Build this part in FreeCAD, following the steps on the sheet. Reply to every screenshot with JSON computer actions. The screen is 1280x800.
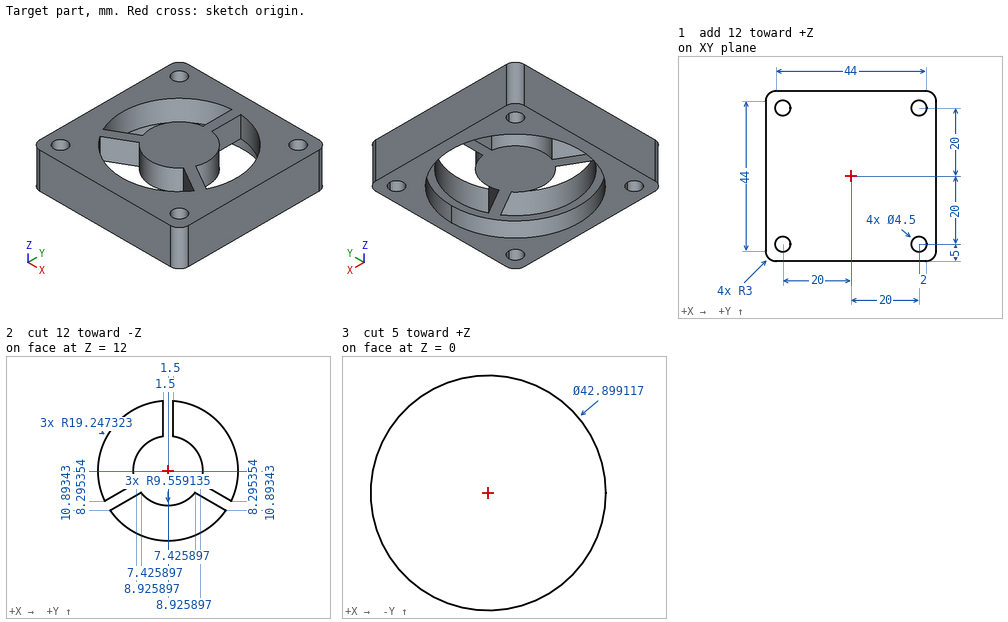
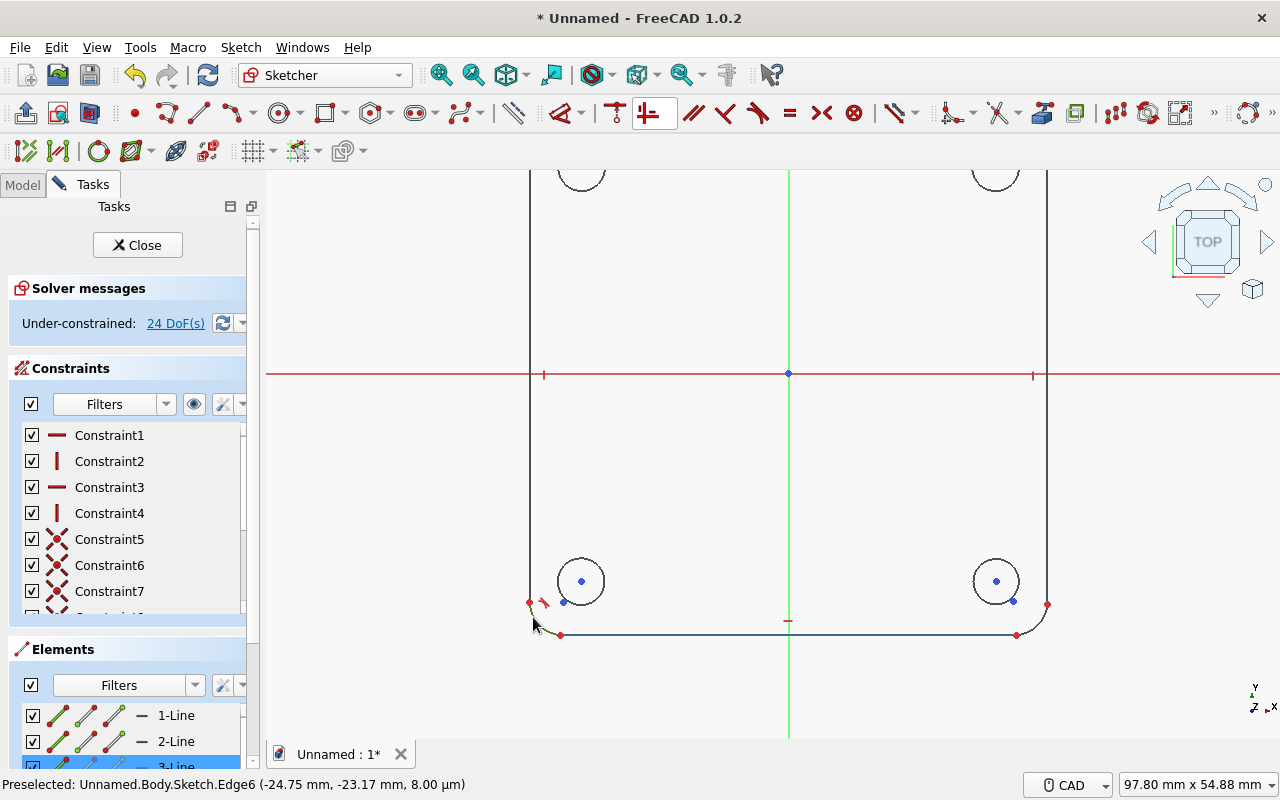
{"action": "left_click", "coordinate": [758, 114]}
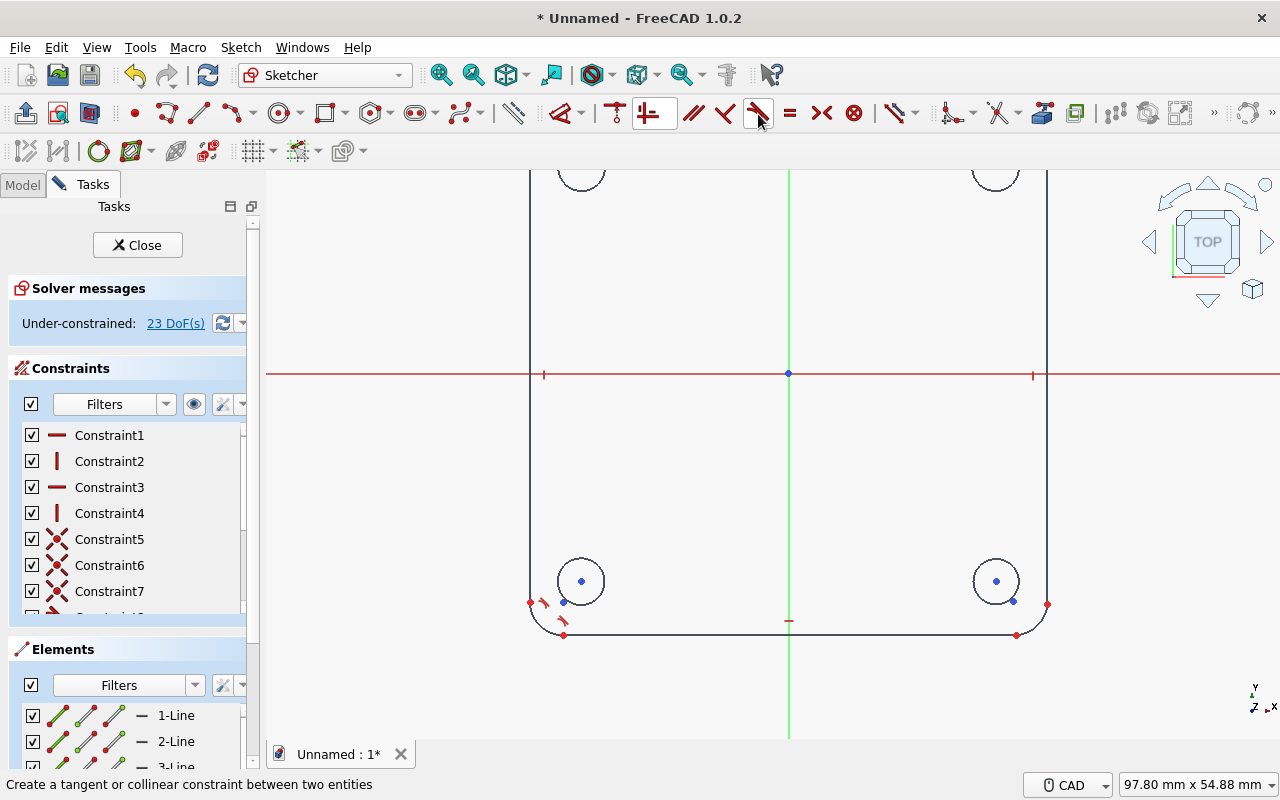
{"action": "left_click", "coordinate": [699, 635]}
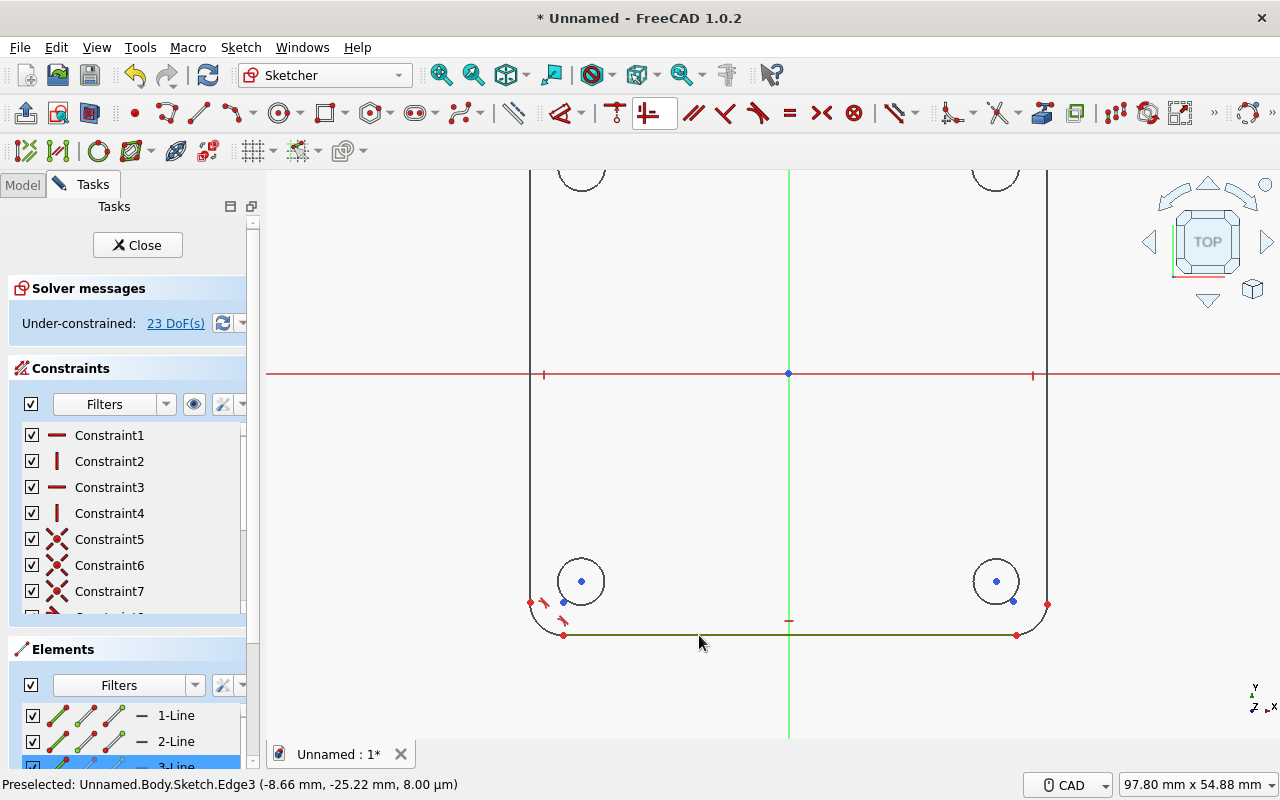
{"action": "left_click", "coordinate": [1030, 631]}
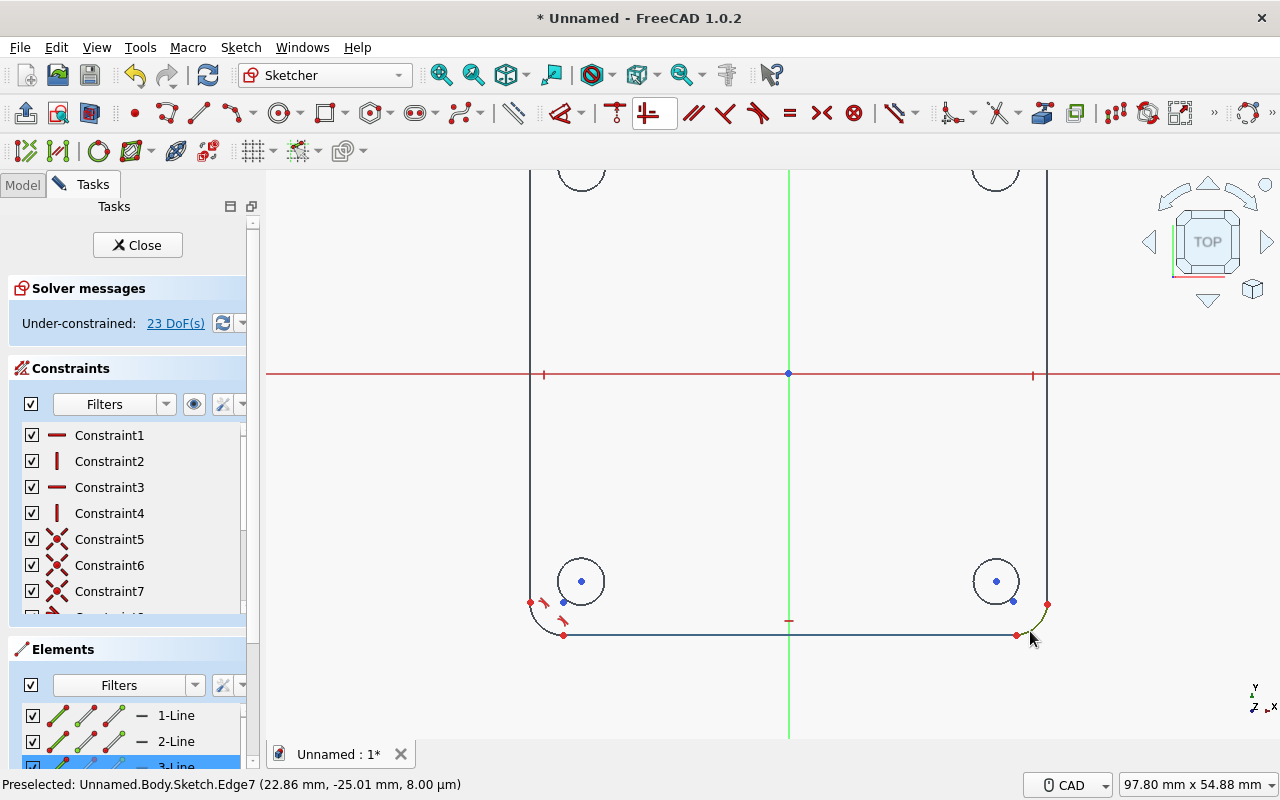
{"action": "left_click", "coordinate": [758, 114]}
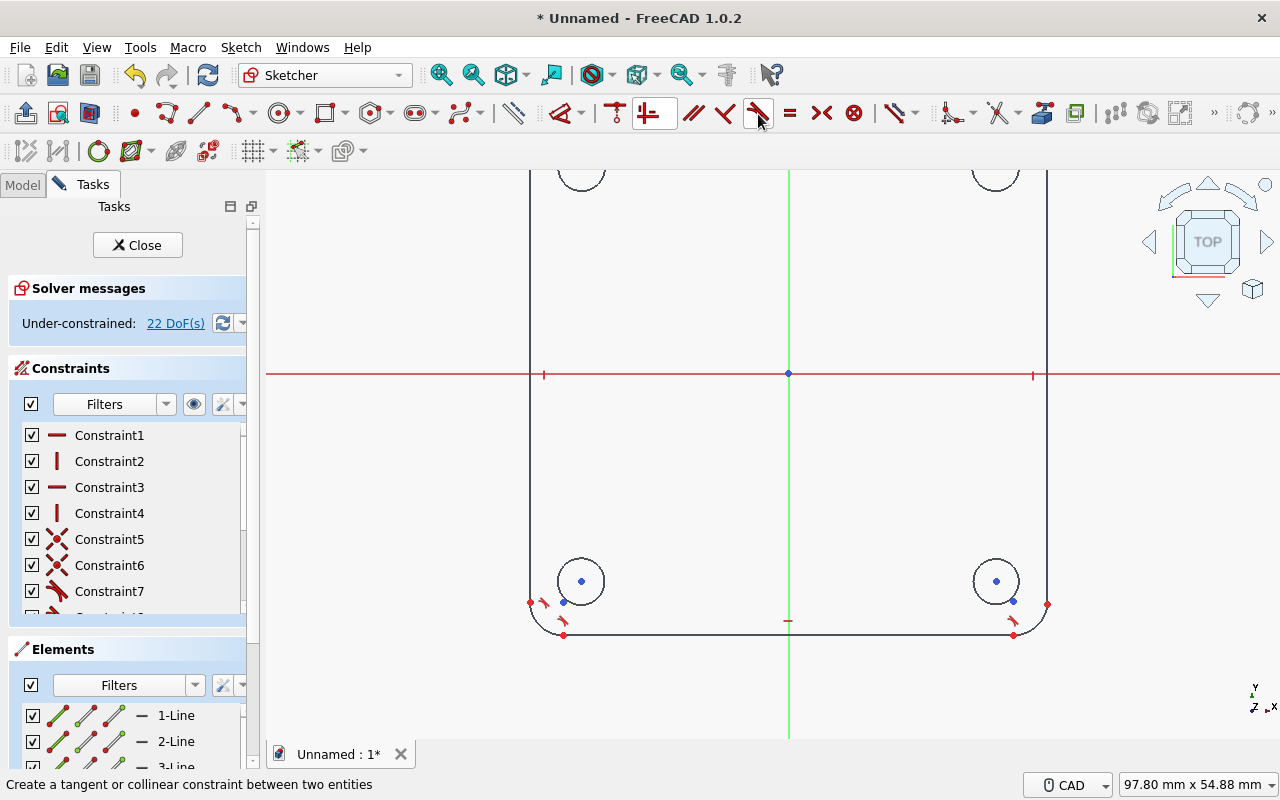
{"action": "left_click", "coordinate": [1047, 467]}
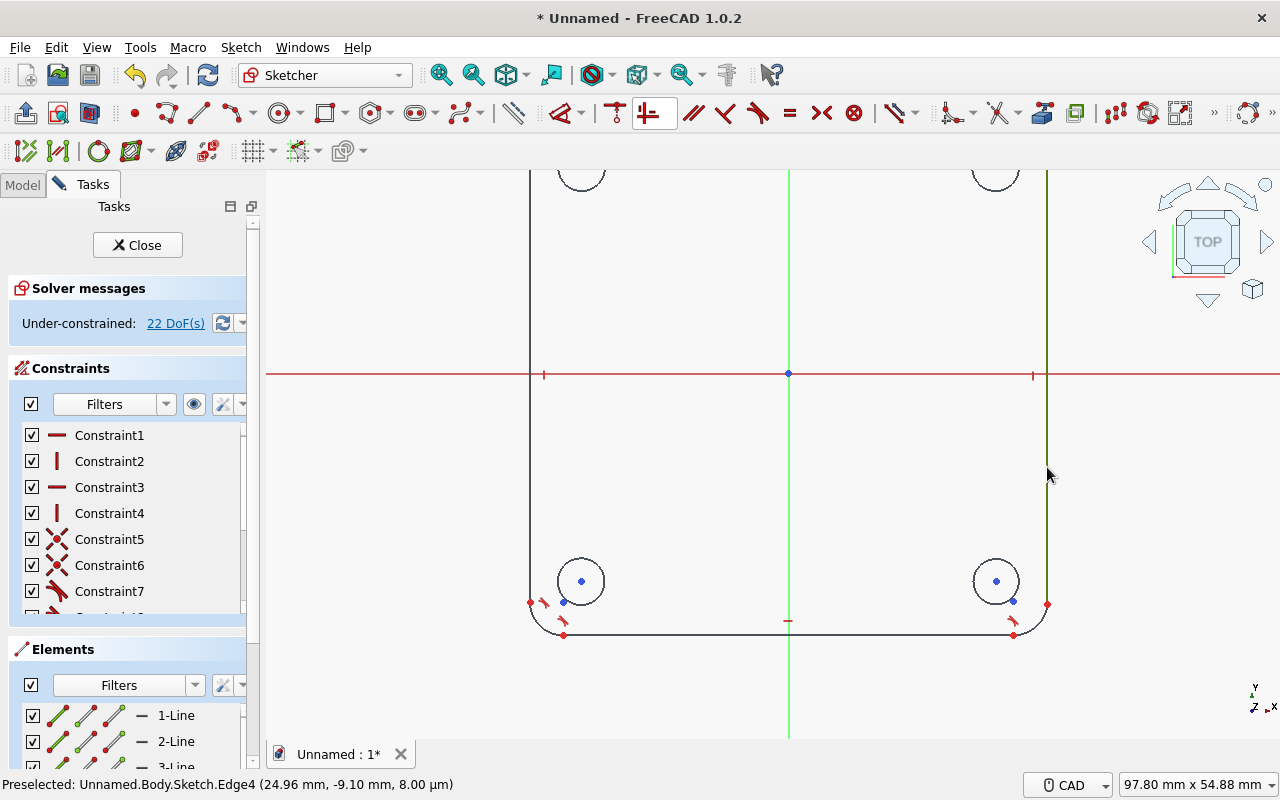
{"action": "left_click", "coordinate": [1028, 632]}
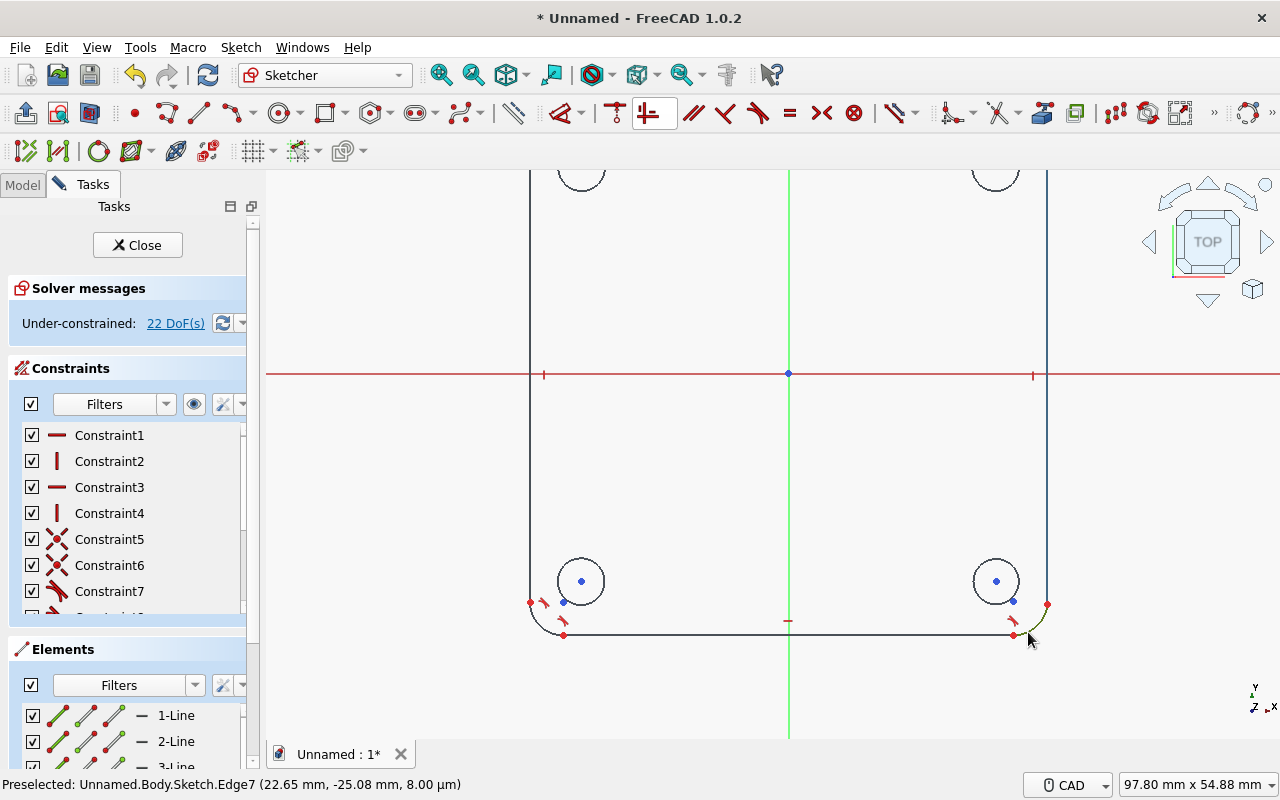
{"action": "left_click", "coordinate": [758, 114]}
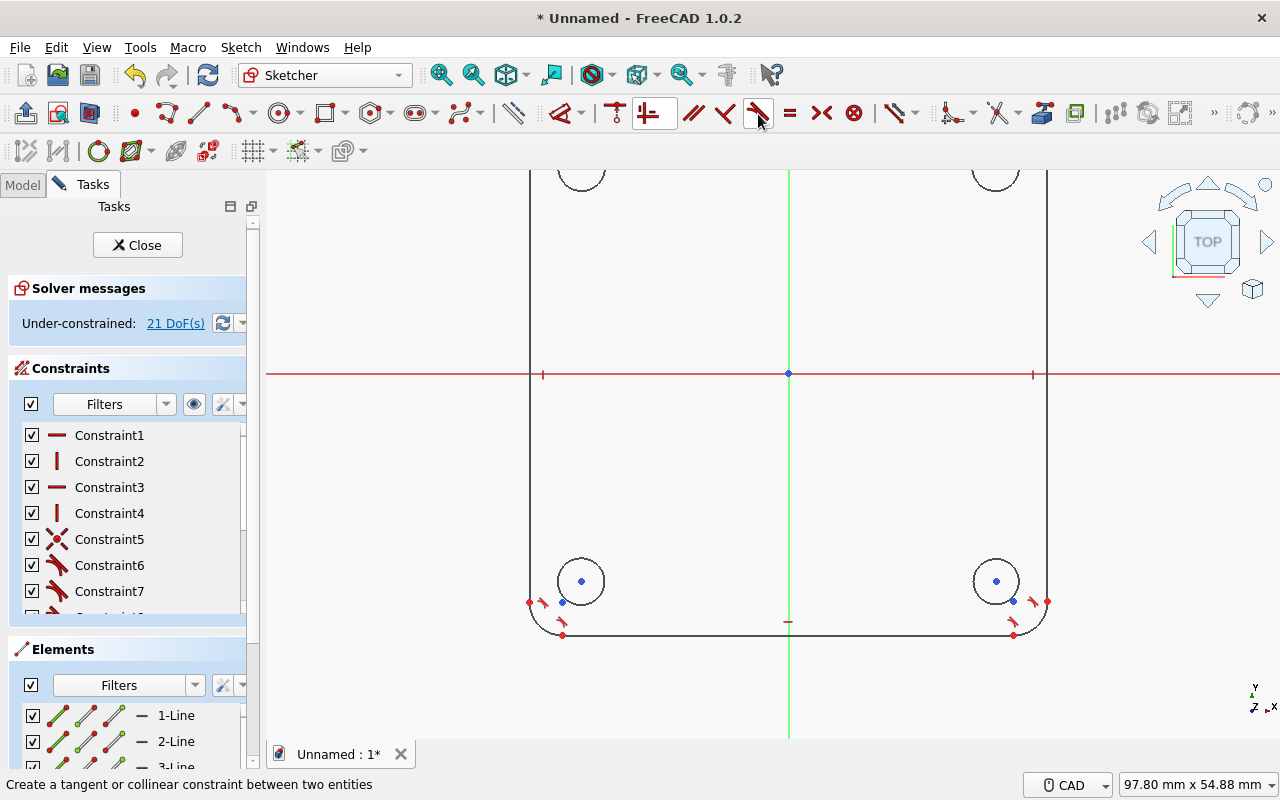
{"action": "left_click", "coordinate": [1047, 465]}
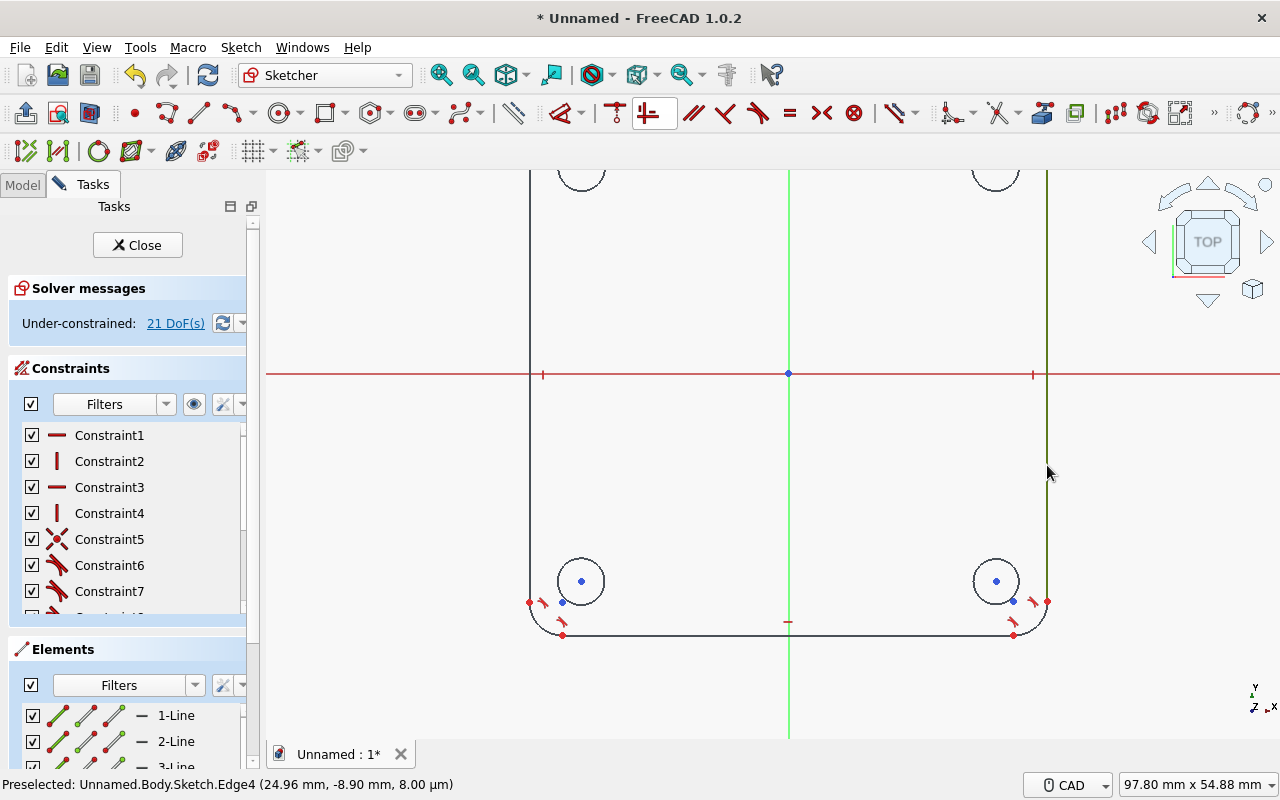
{"action": "scroll", "coordinate": [533, 619], "scroll_direction": "down", "scroll_amount": 2}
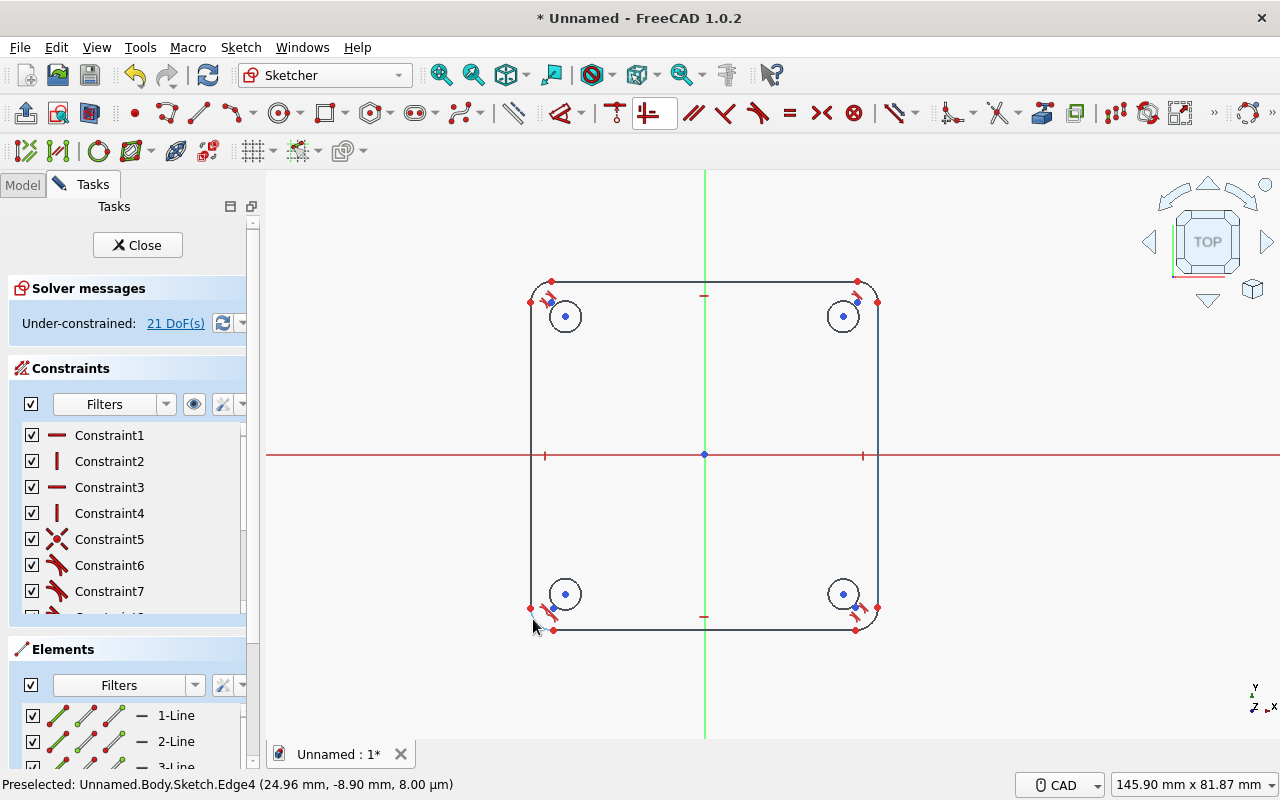
{"action": "scroll", "coordinate": [876, 293], "scroll_direction": "up", "scroll_amount": 2}